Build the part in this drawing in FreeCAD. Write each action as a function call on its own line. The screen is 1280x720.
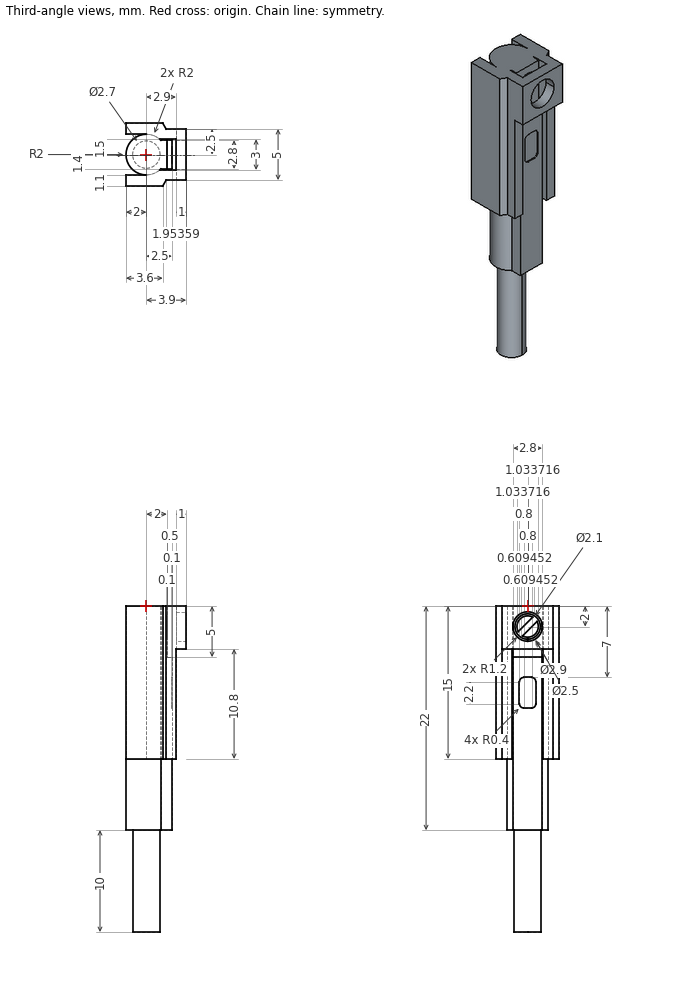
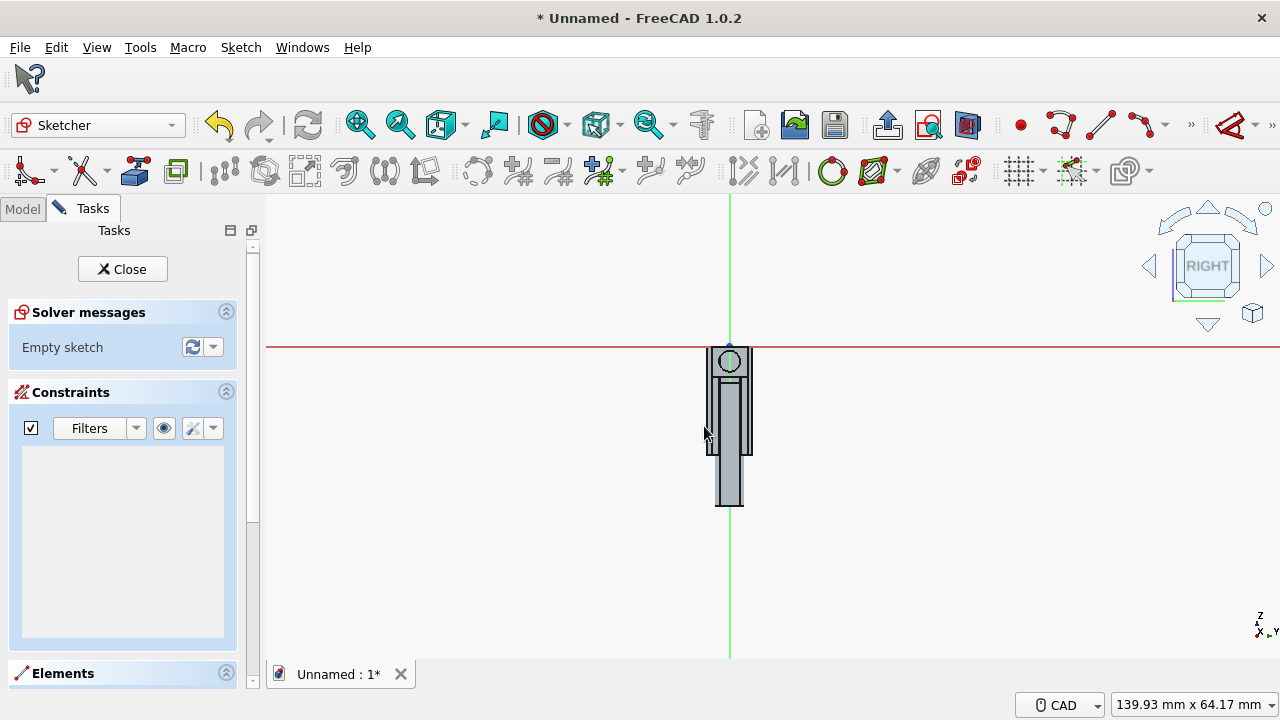
scroll(732, 353, up, 13)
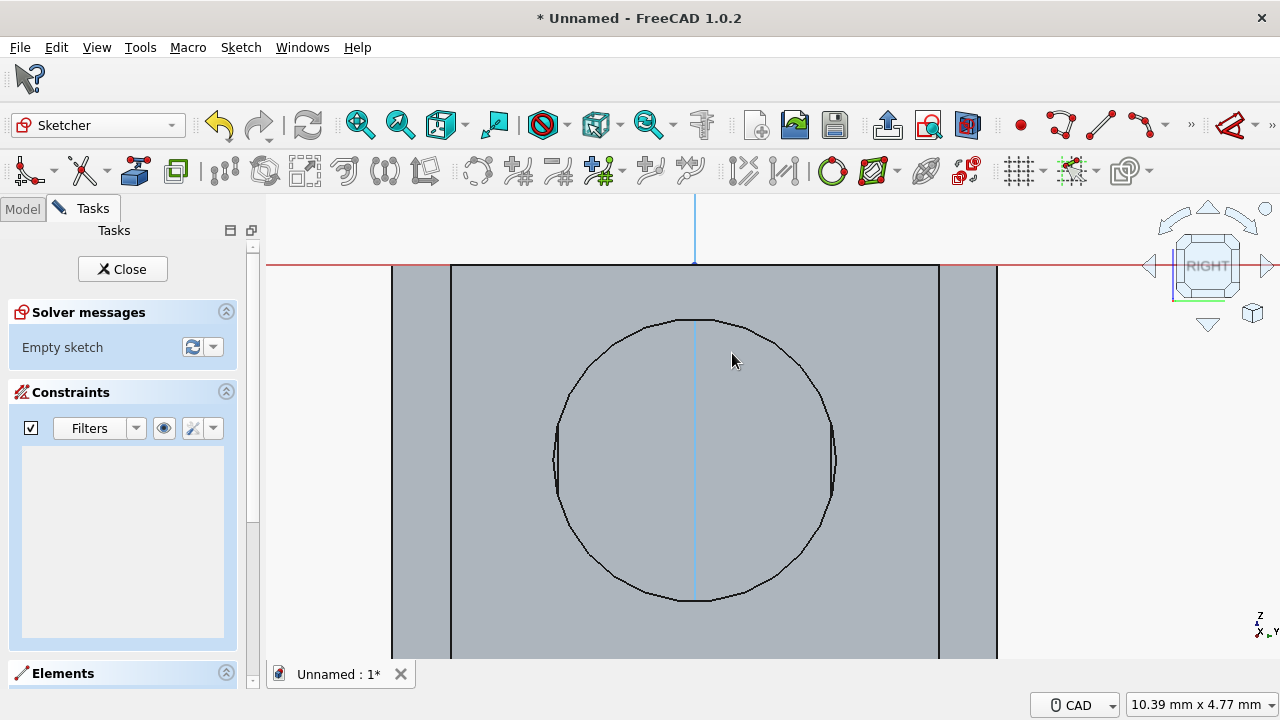
key(g)
key(c)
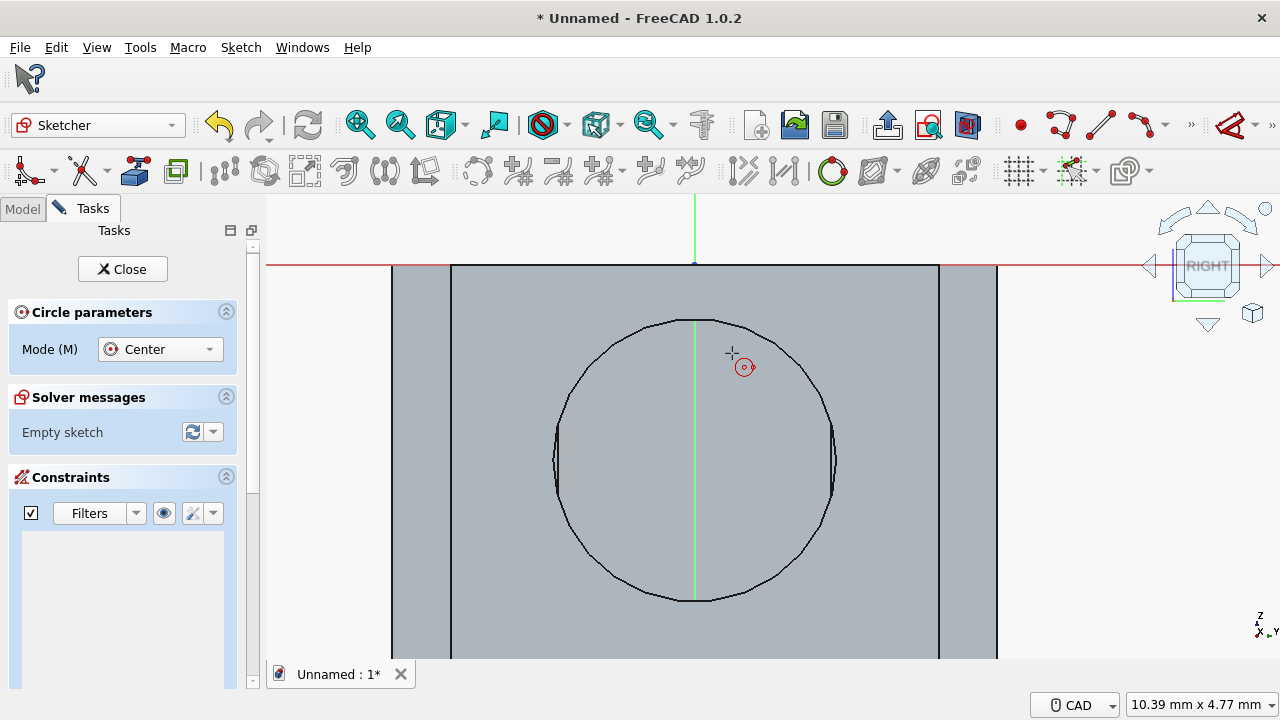
click(695, 460)
click(781, 374)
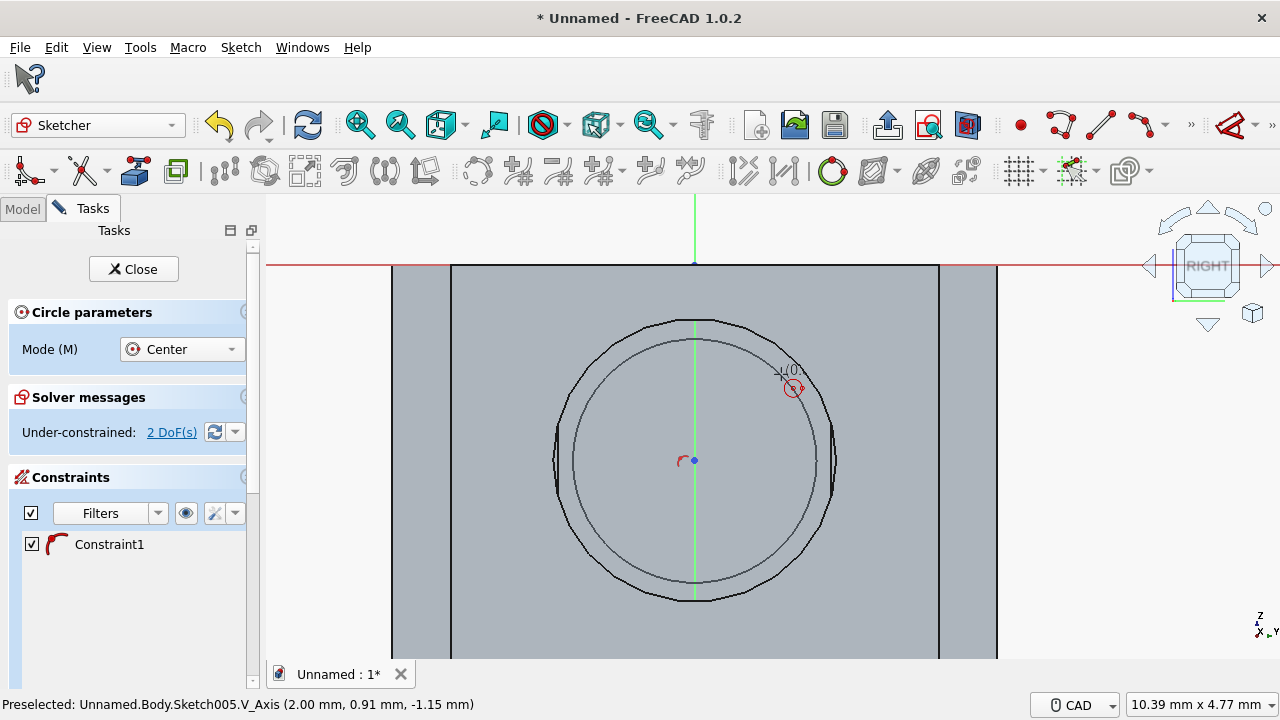
click(695, 461)
click(767, 388)
key(Escape)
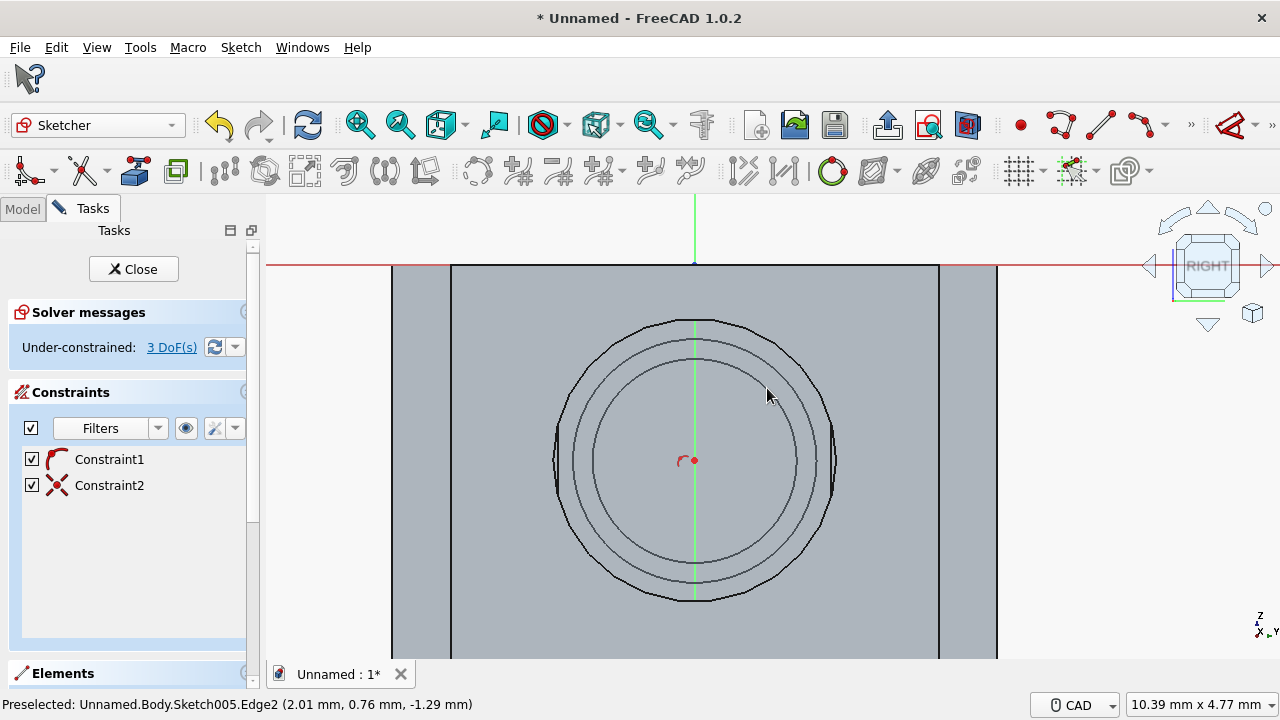
click(1230, 126)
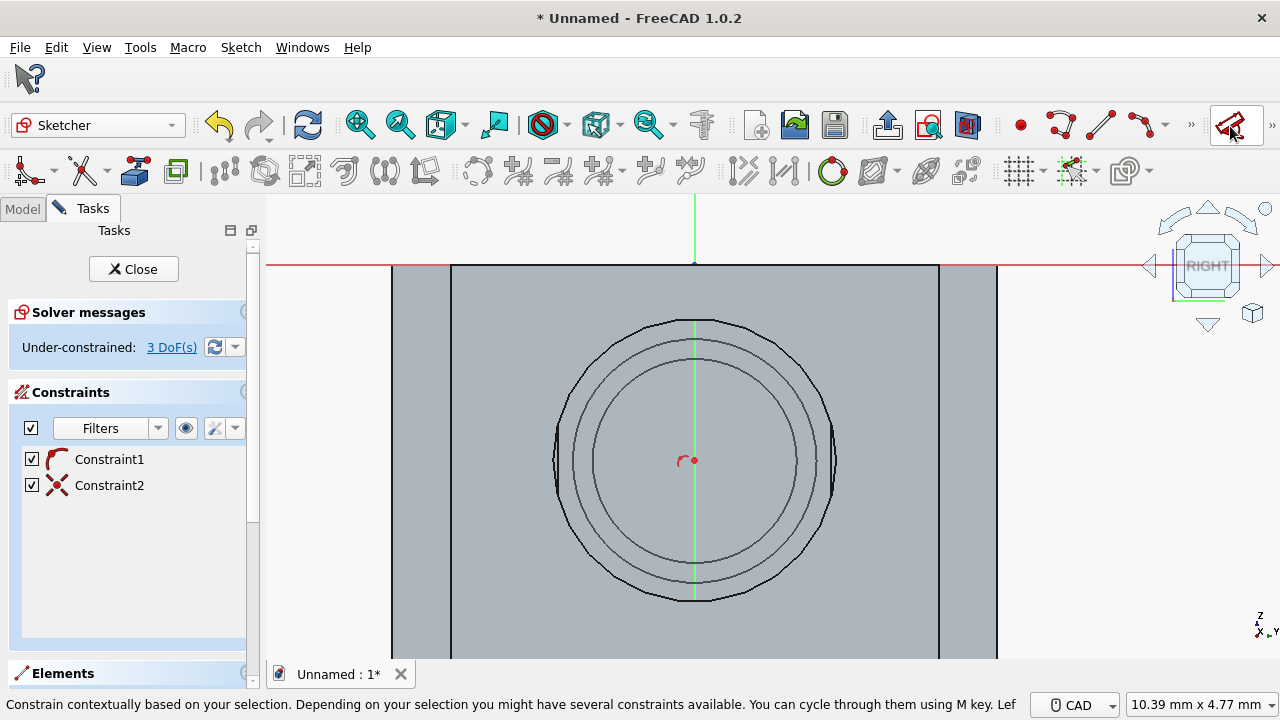
click(781, 375)
click(804, 352)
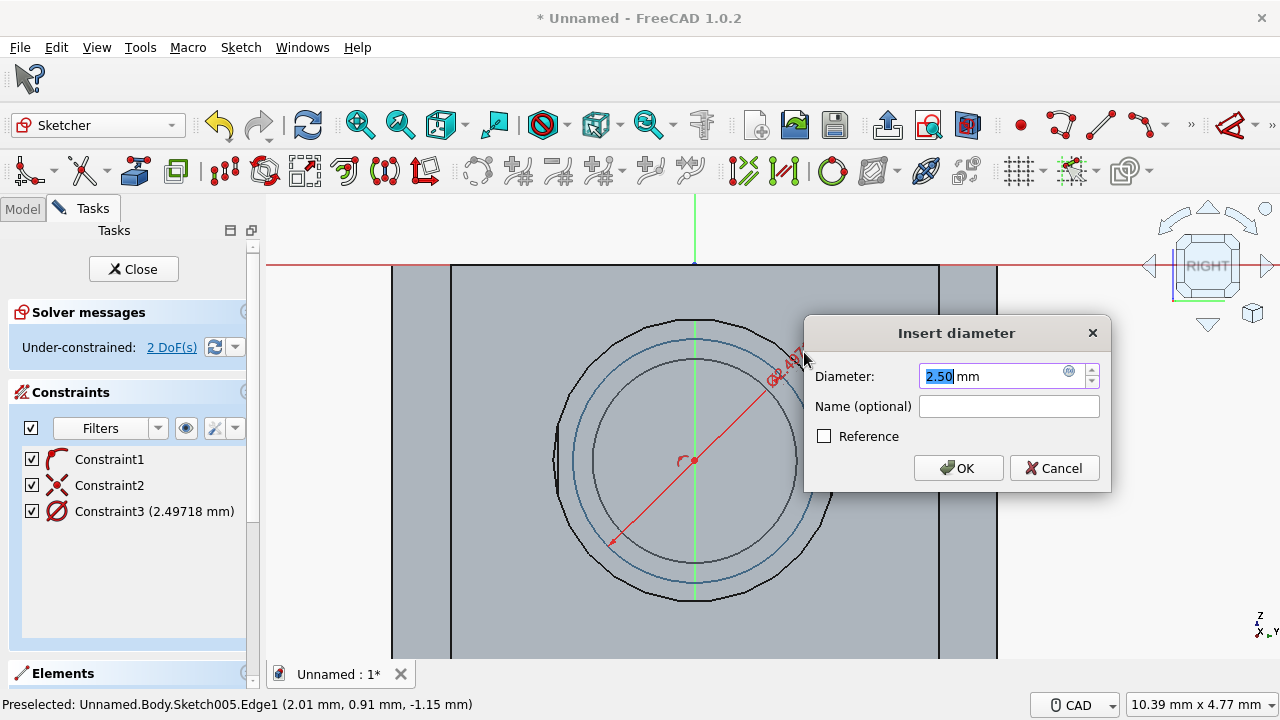
text(2.5)
key(Return)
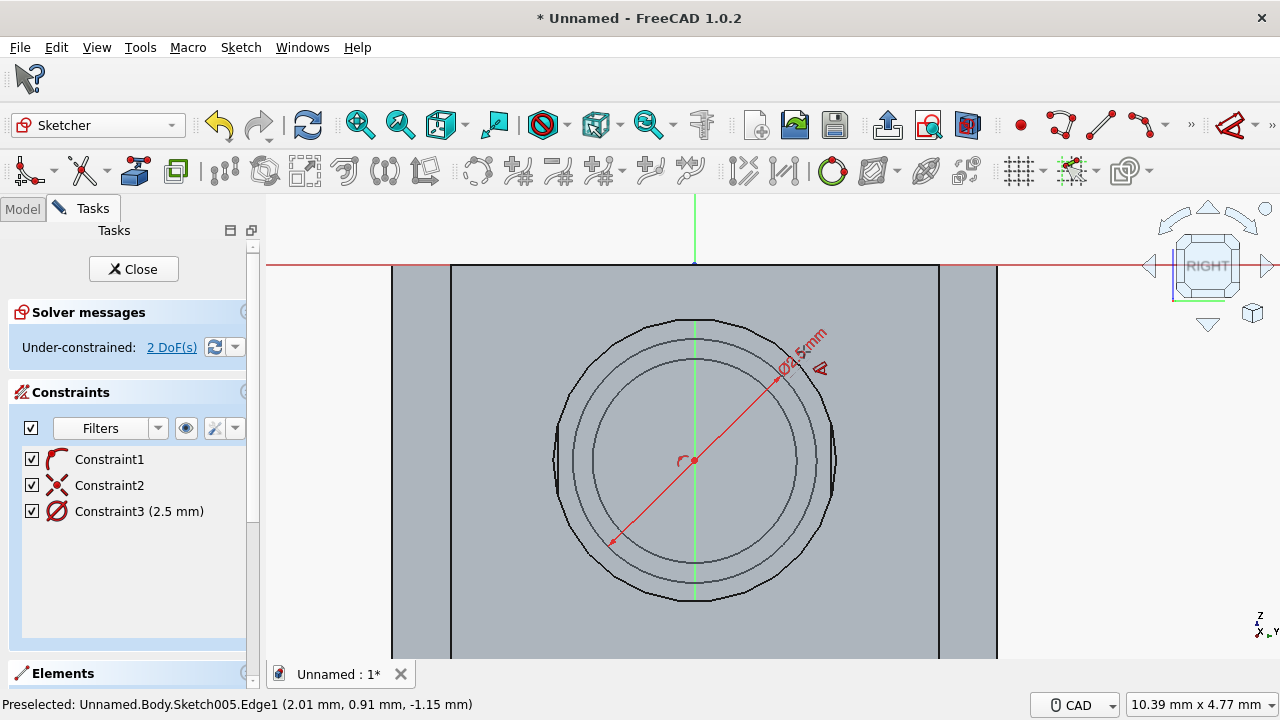
click(767, 389)
click(845, 417)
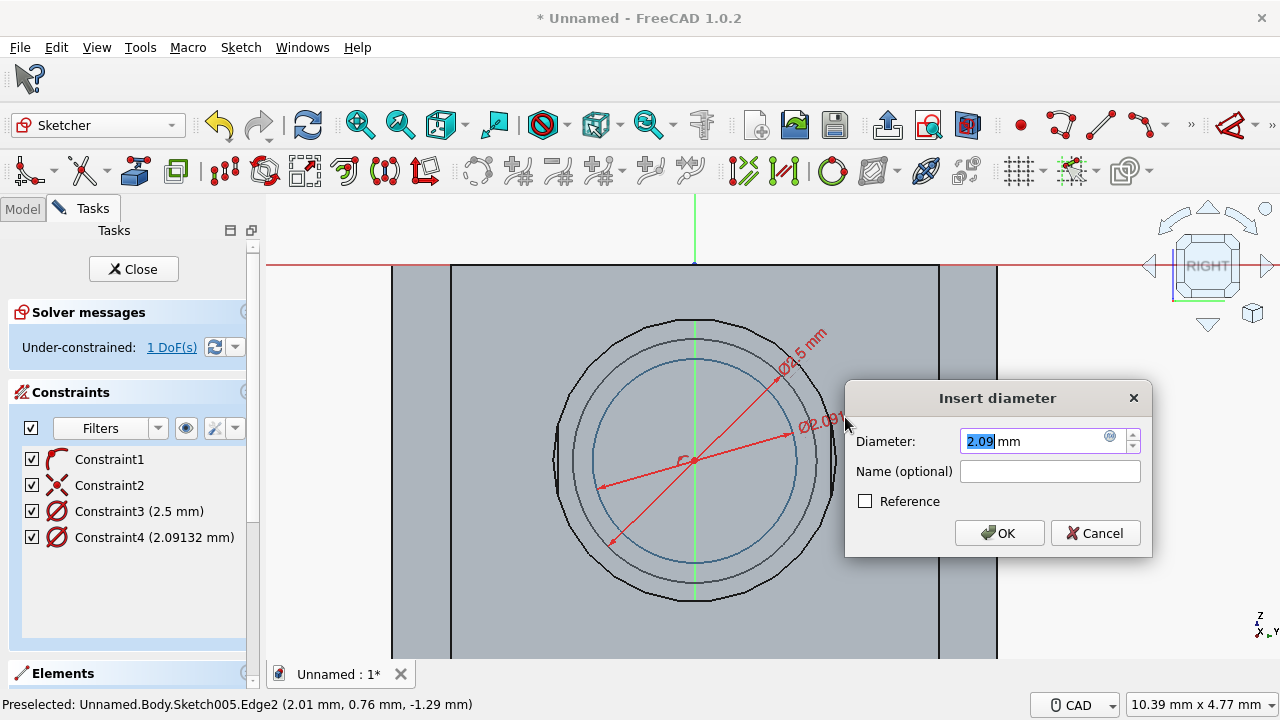
text(2.1)
key(Return)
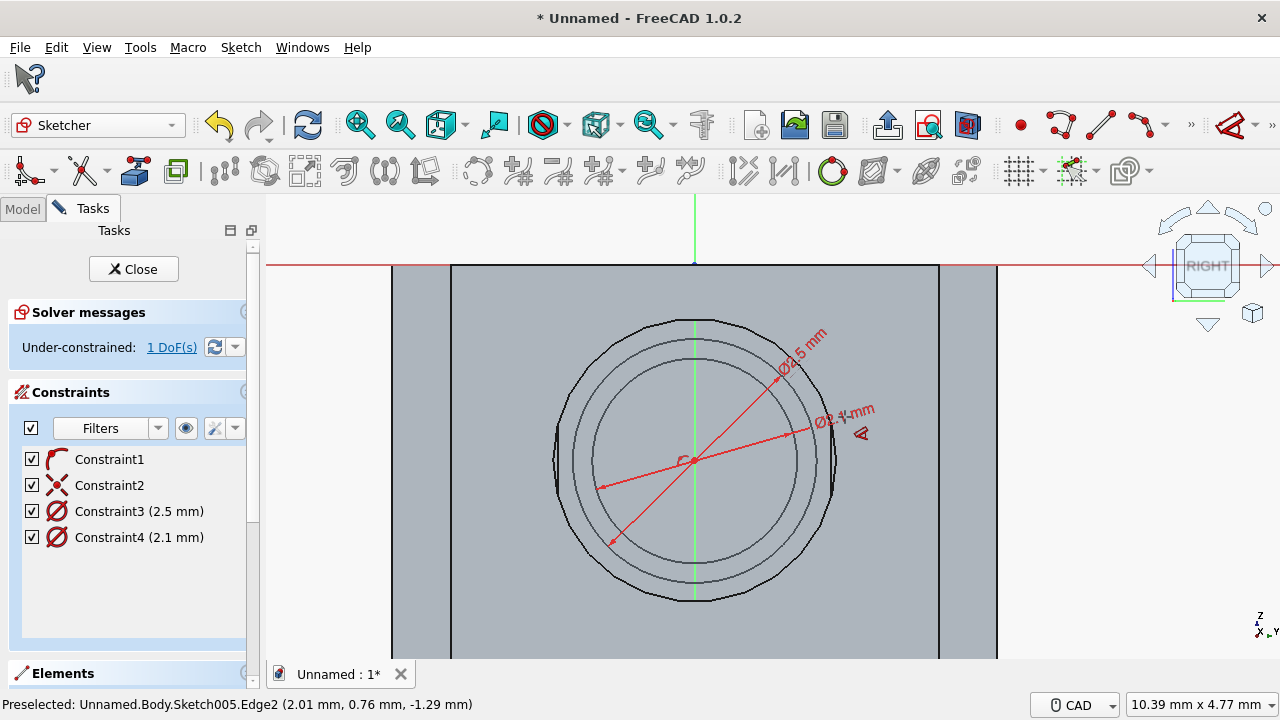
click(695, 461)
click(729, 318)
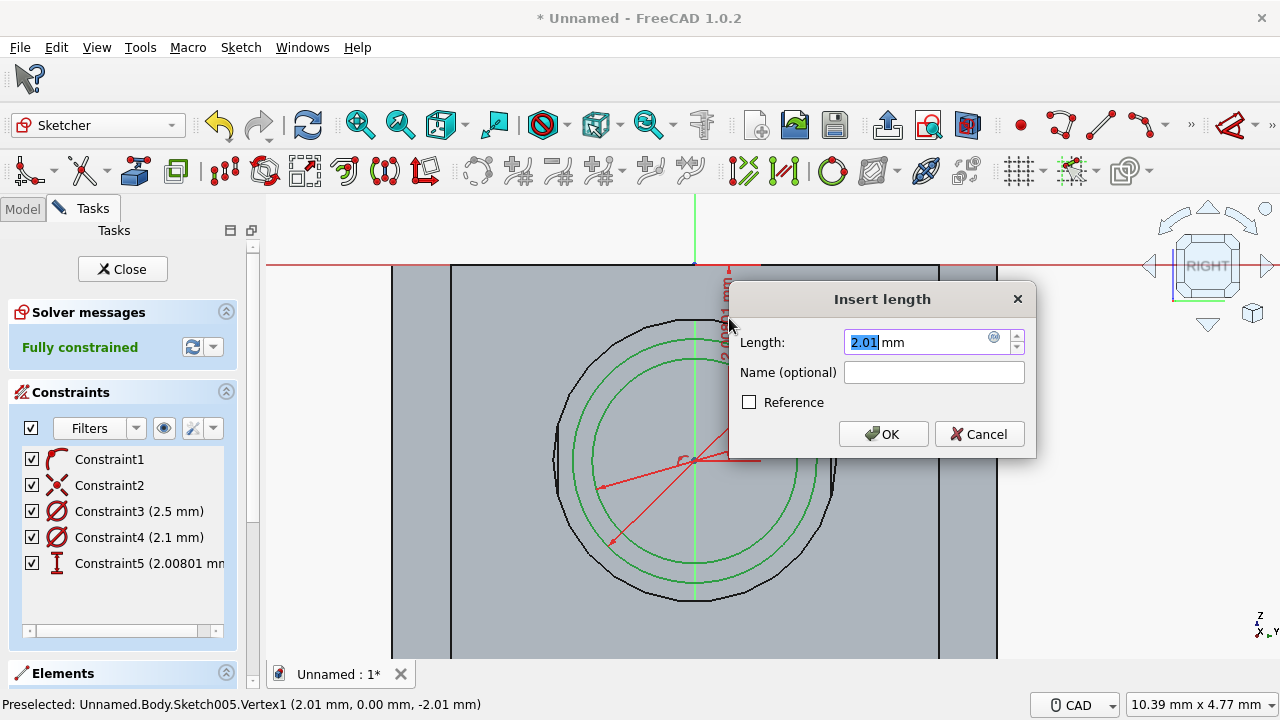
text(2)
key(Return)
key(Escape)